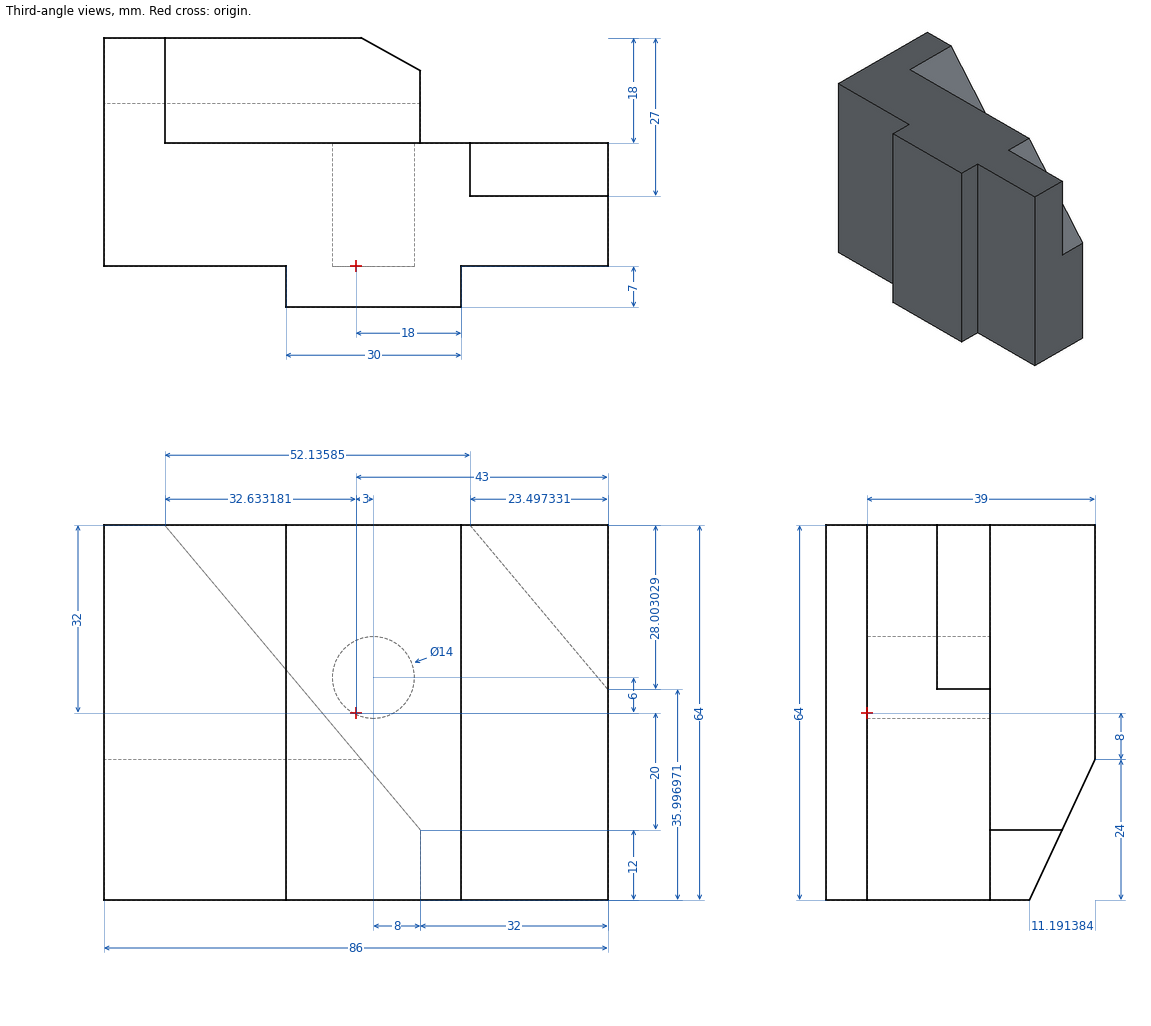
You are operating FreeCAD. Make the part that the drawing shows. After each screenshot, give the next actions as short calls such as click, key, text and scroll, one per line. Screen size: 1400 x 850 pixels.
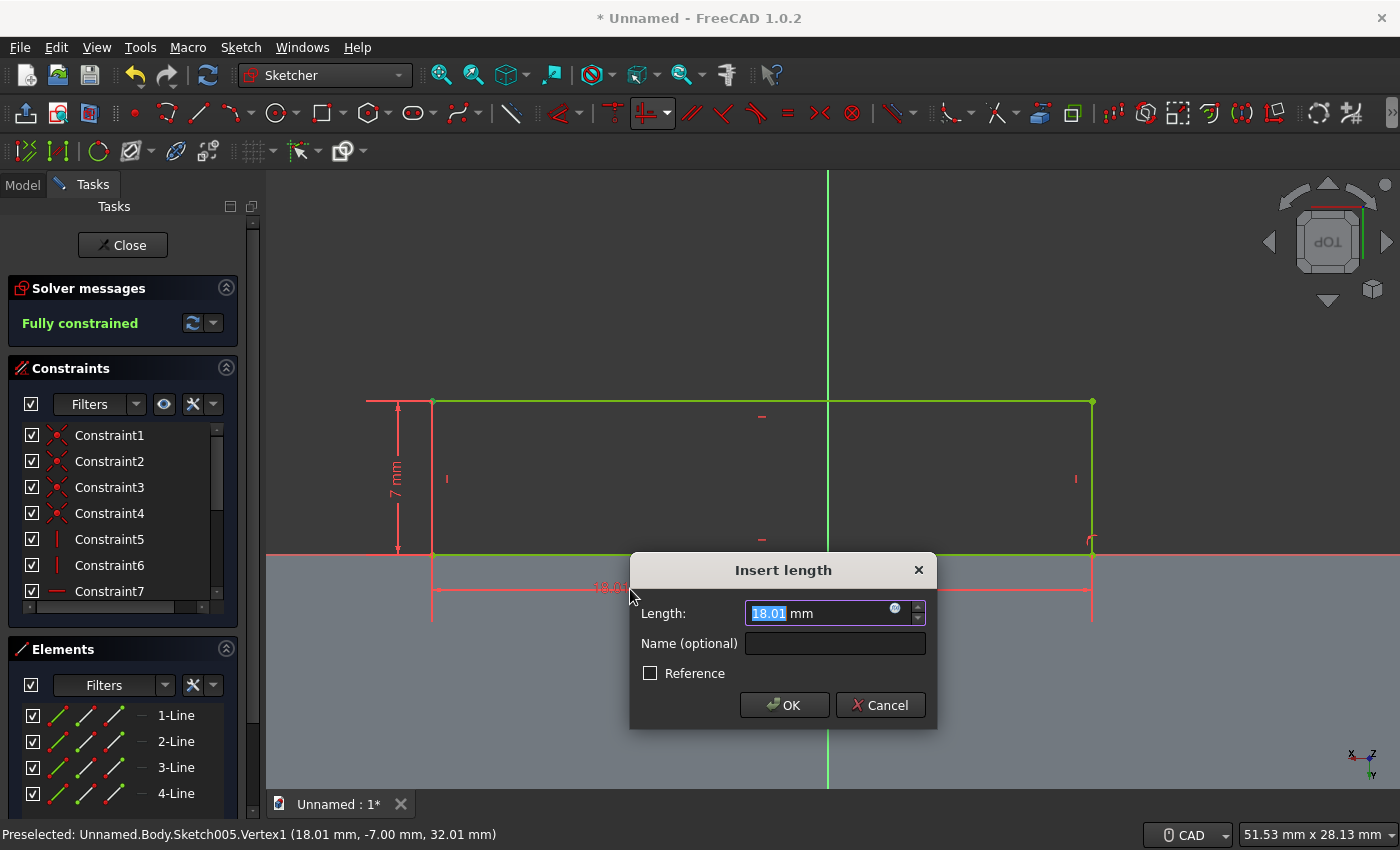
text(18)
key(Return)
key(Escape)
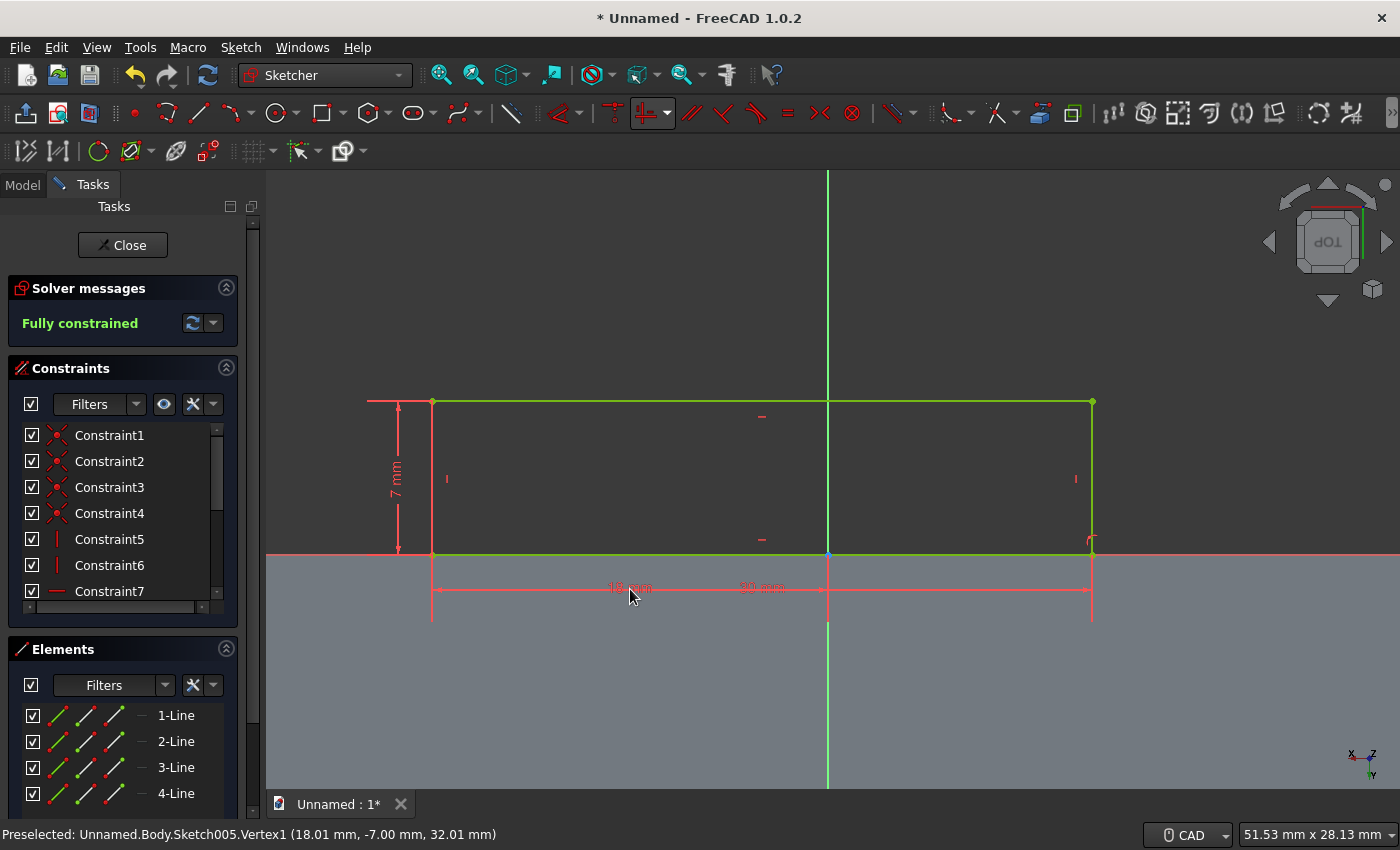
click(123, 245)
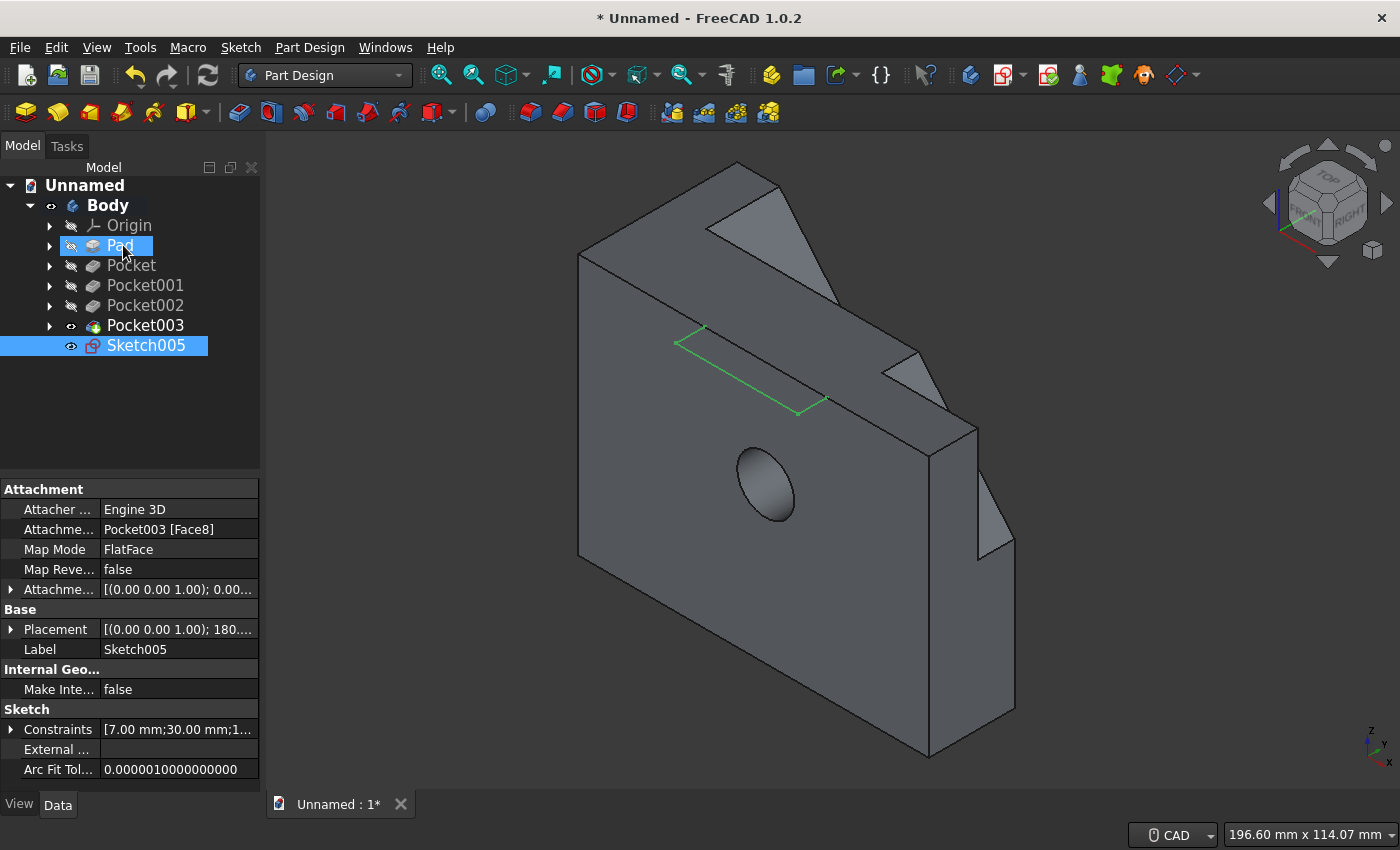
click(26, 112)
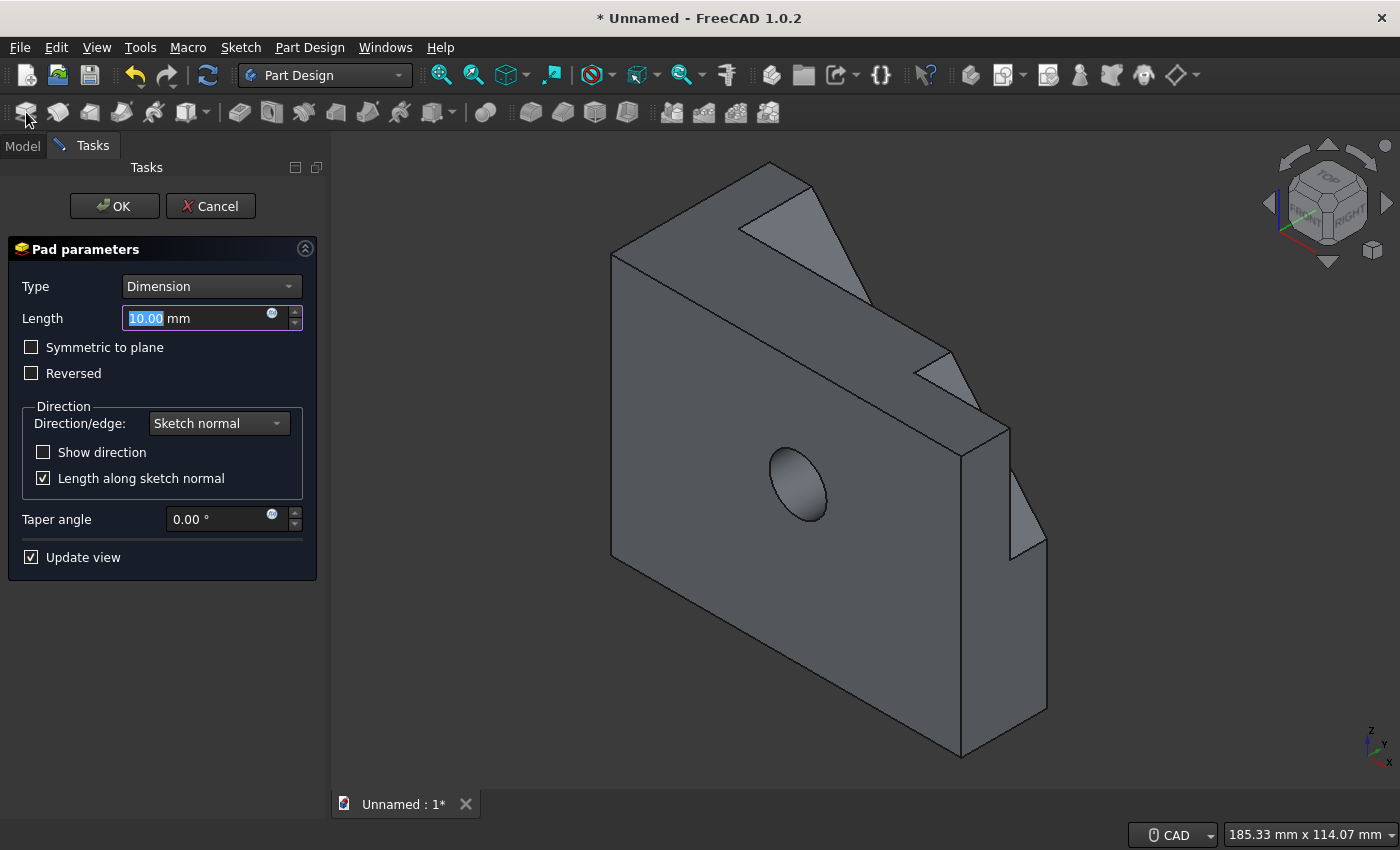
text(64)
key(Tab)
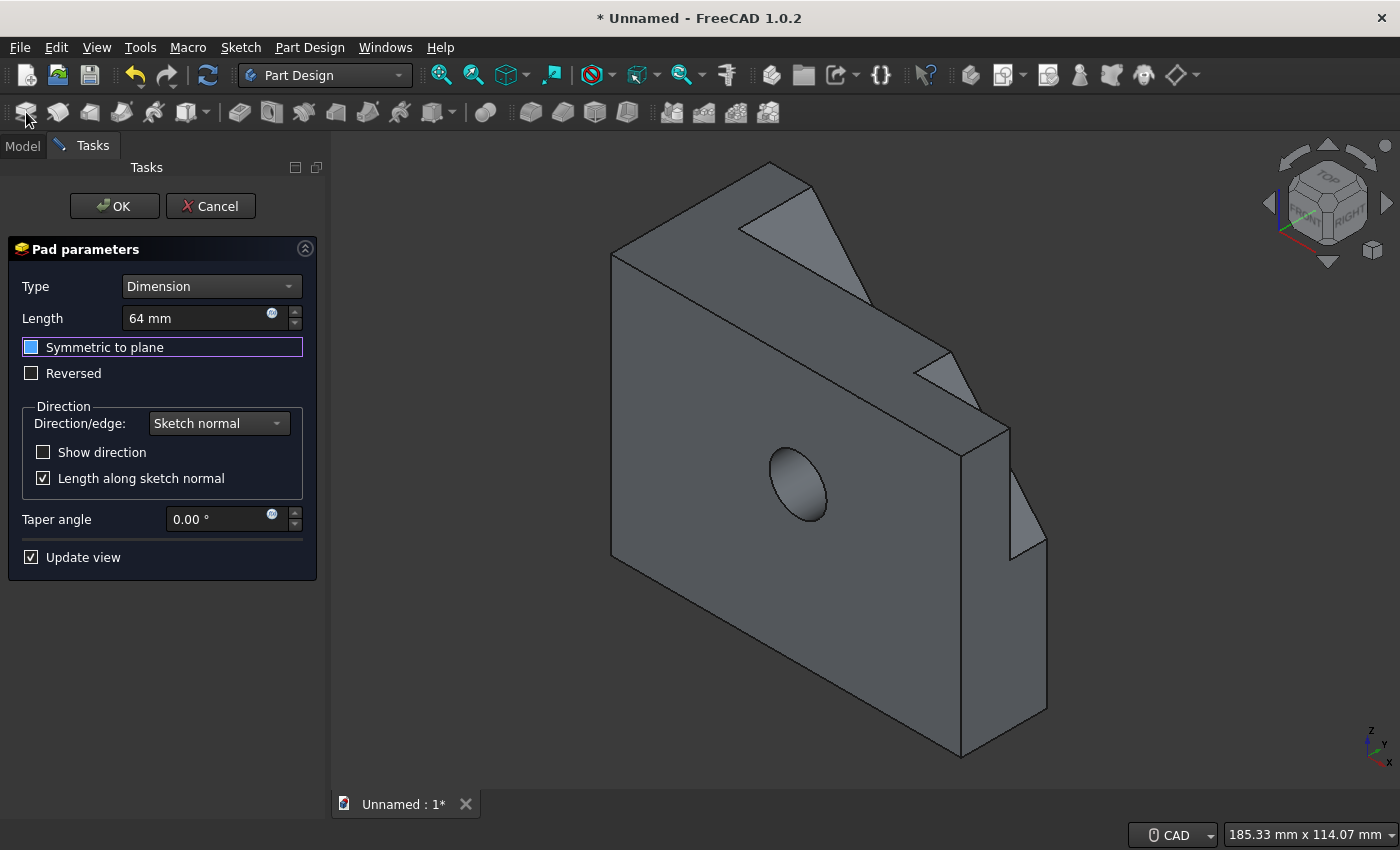
click(30, 373)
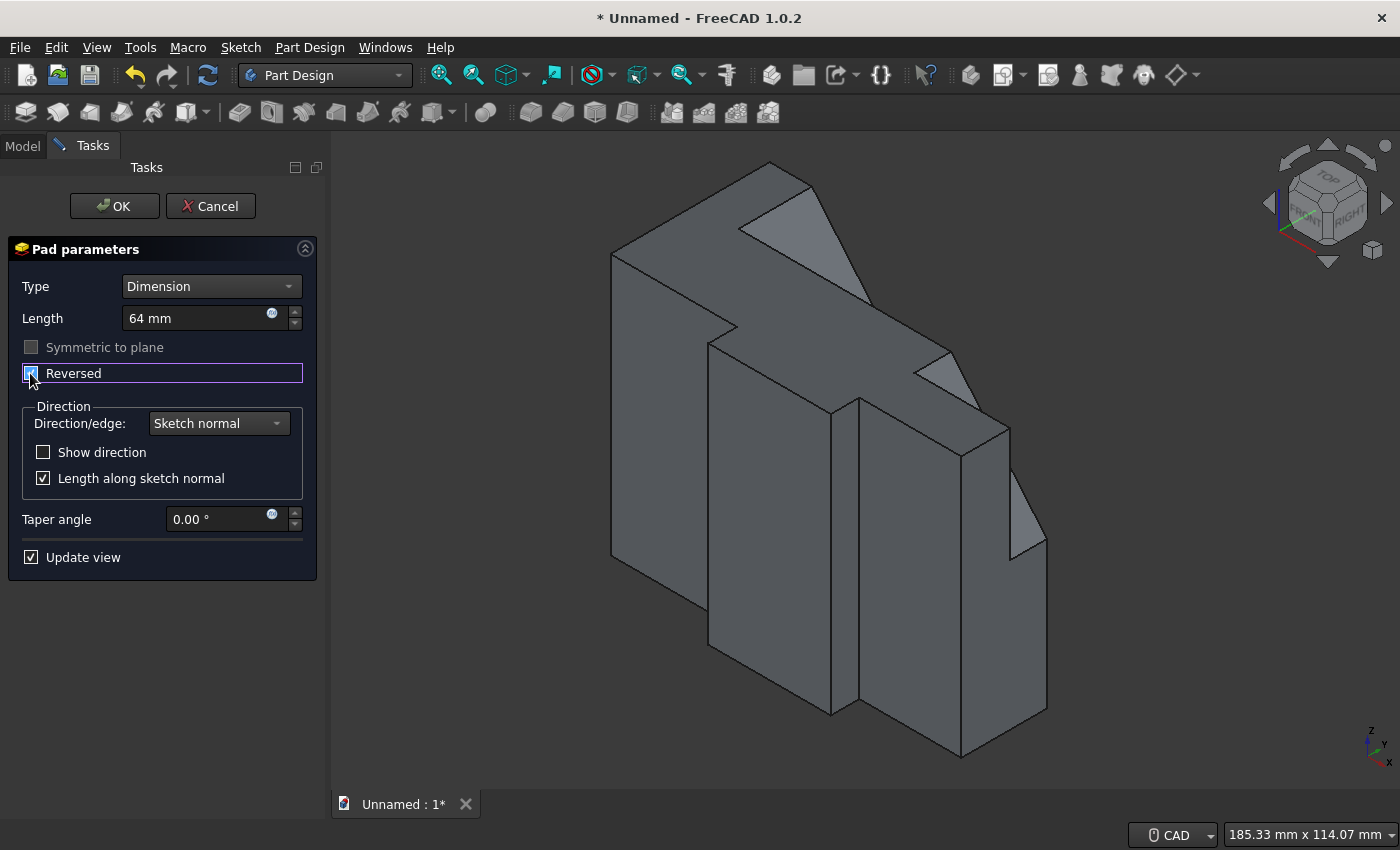
click(115, 206)